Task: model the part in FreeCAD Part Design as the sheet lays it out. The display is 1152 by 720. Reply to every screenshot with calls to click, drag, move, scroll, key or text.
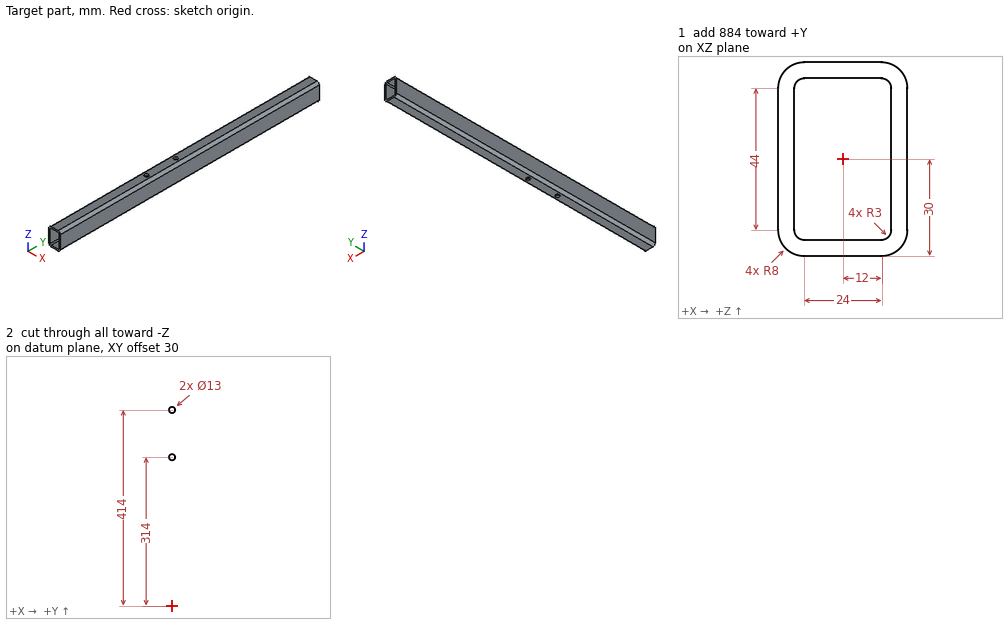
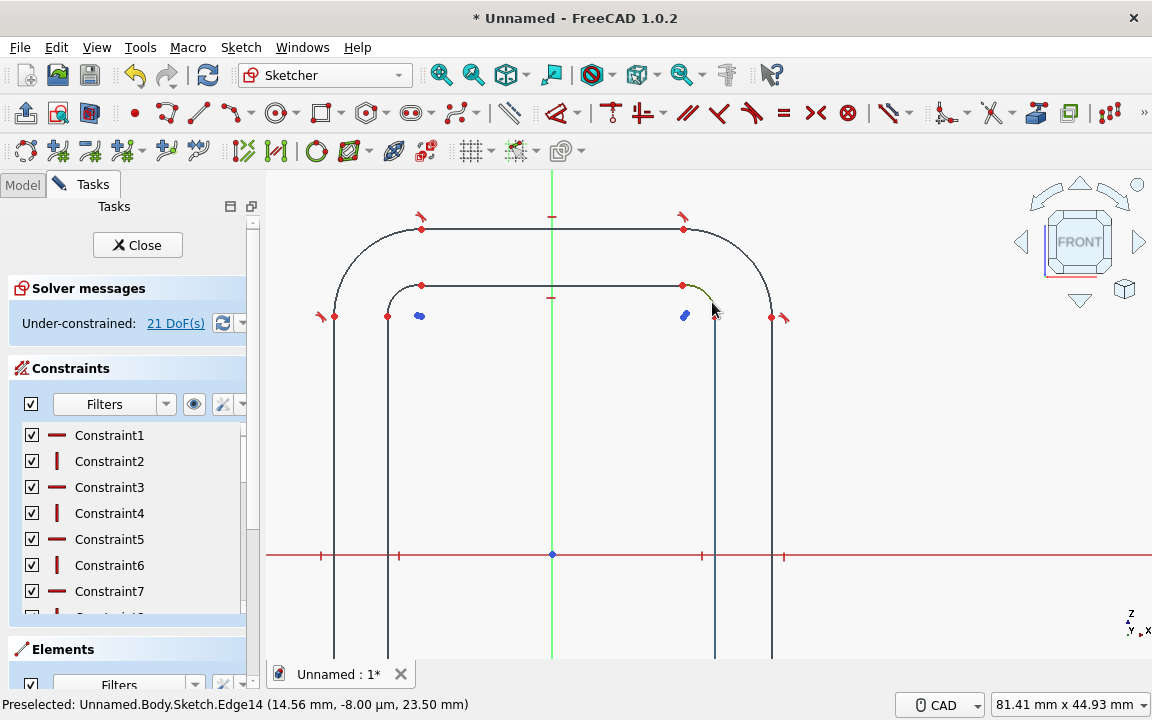
key(t)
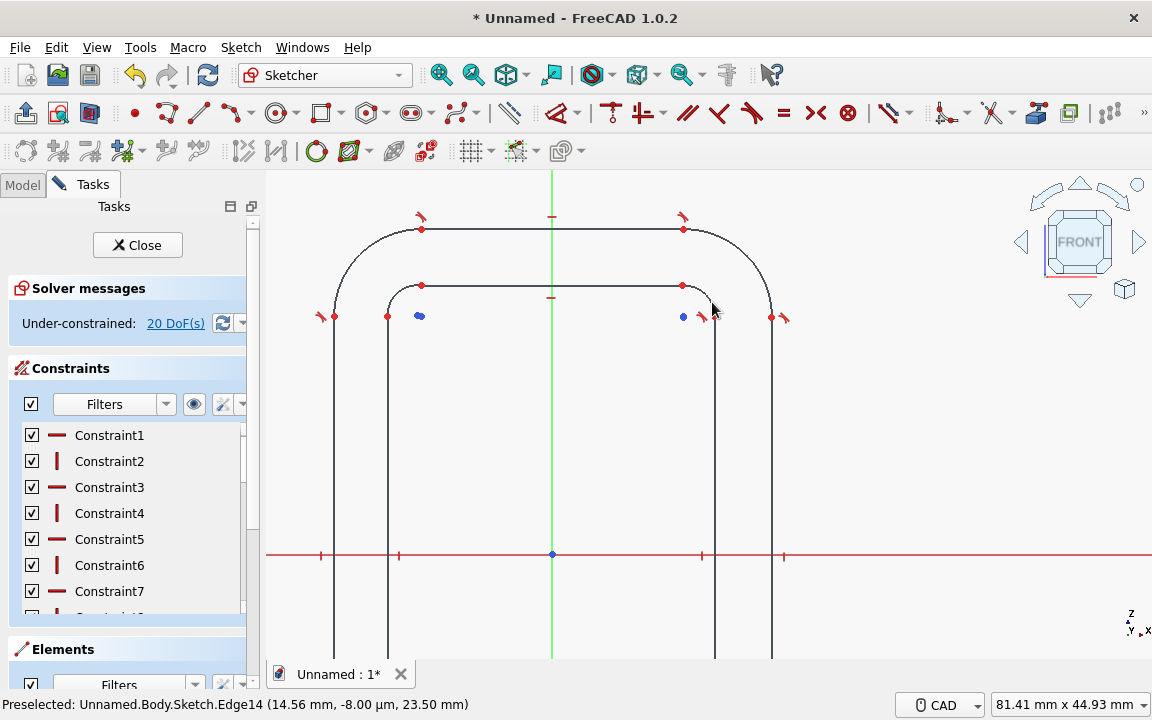
click(604, 286)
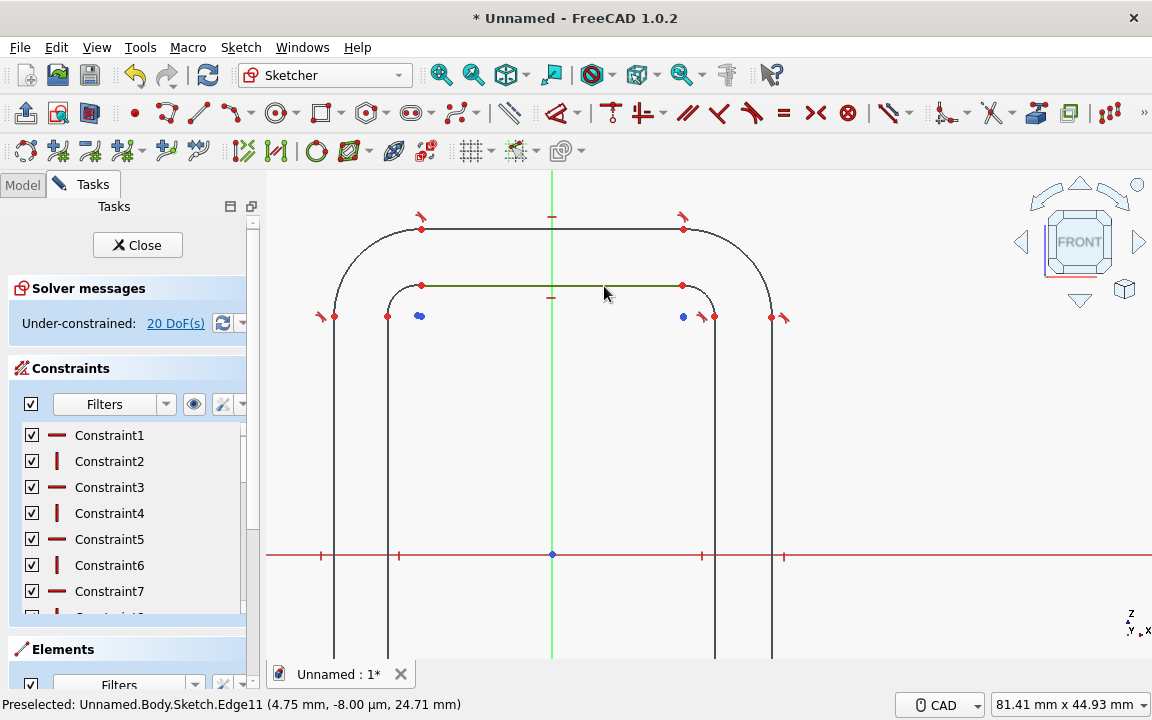
click(711, 302)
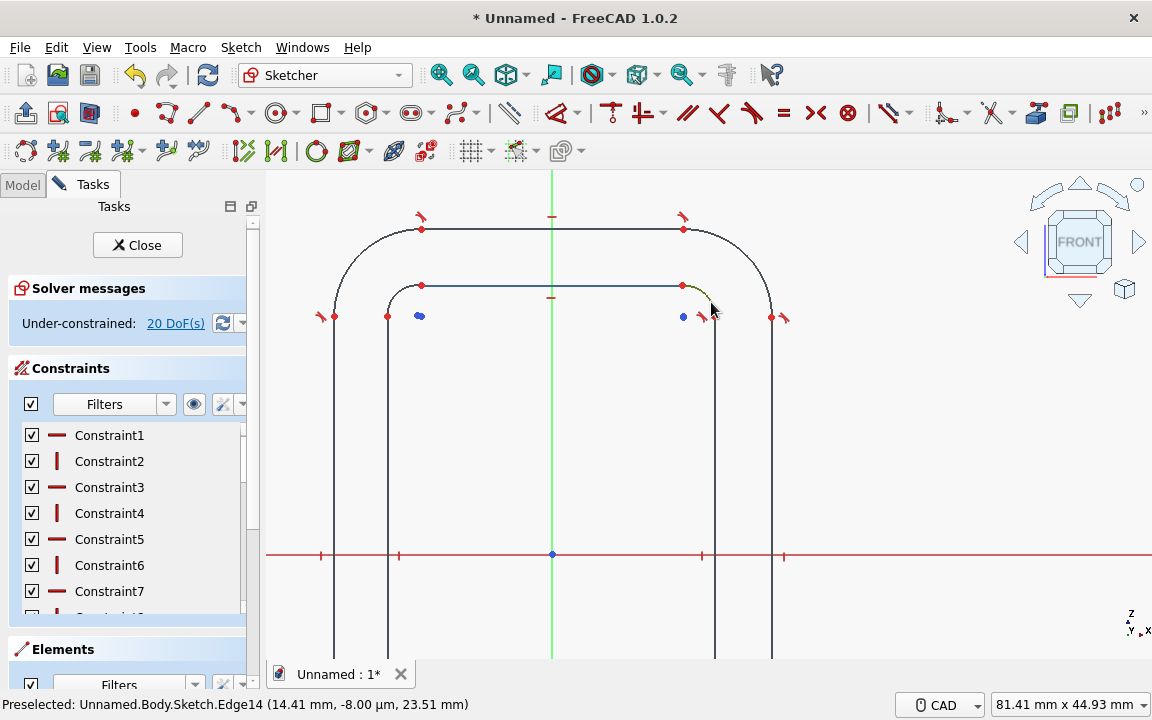
key(t)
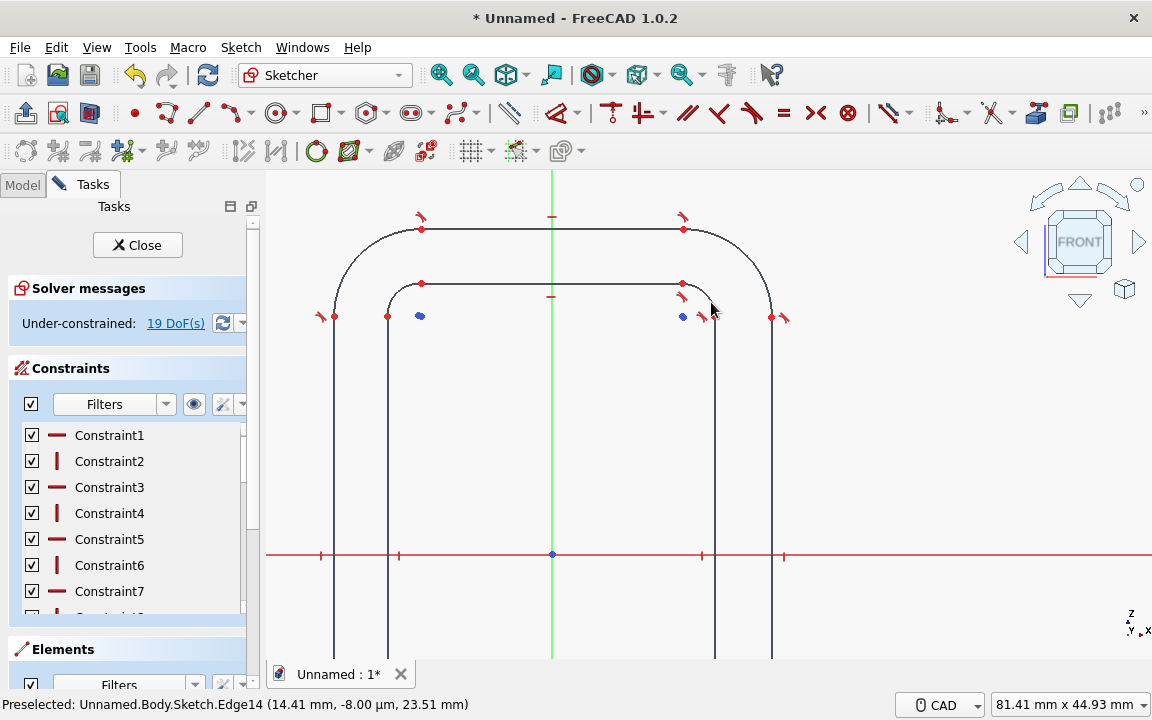
click(604, 284)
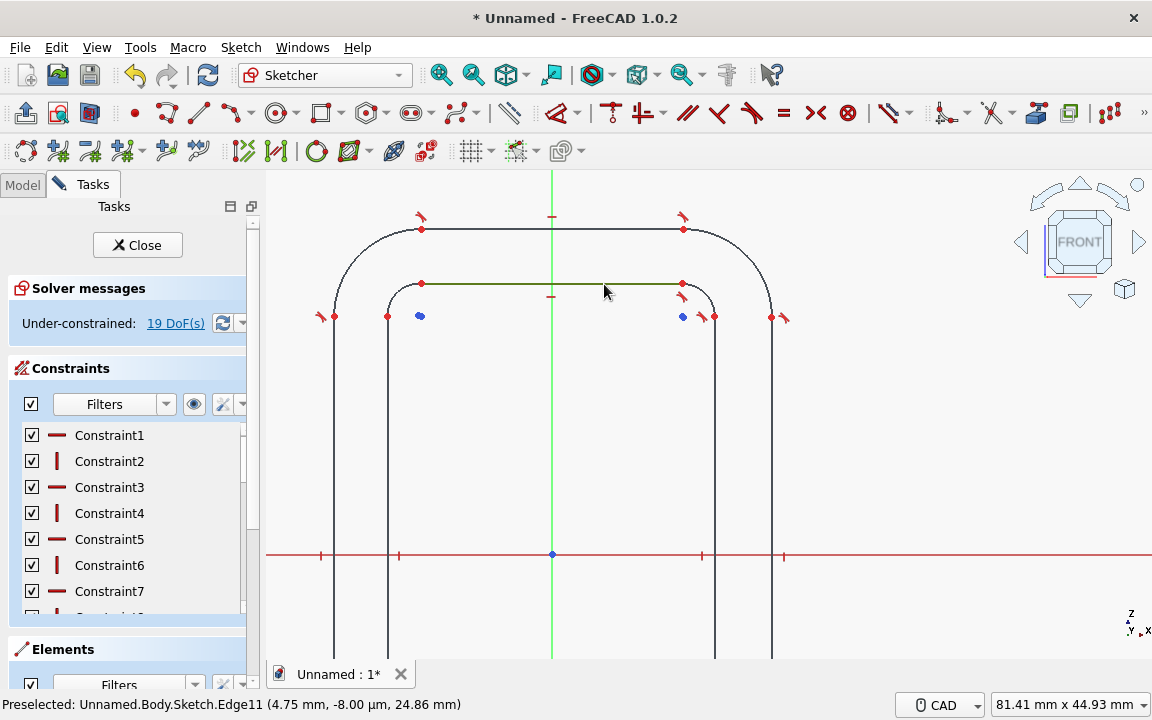
click(406, 287)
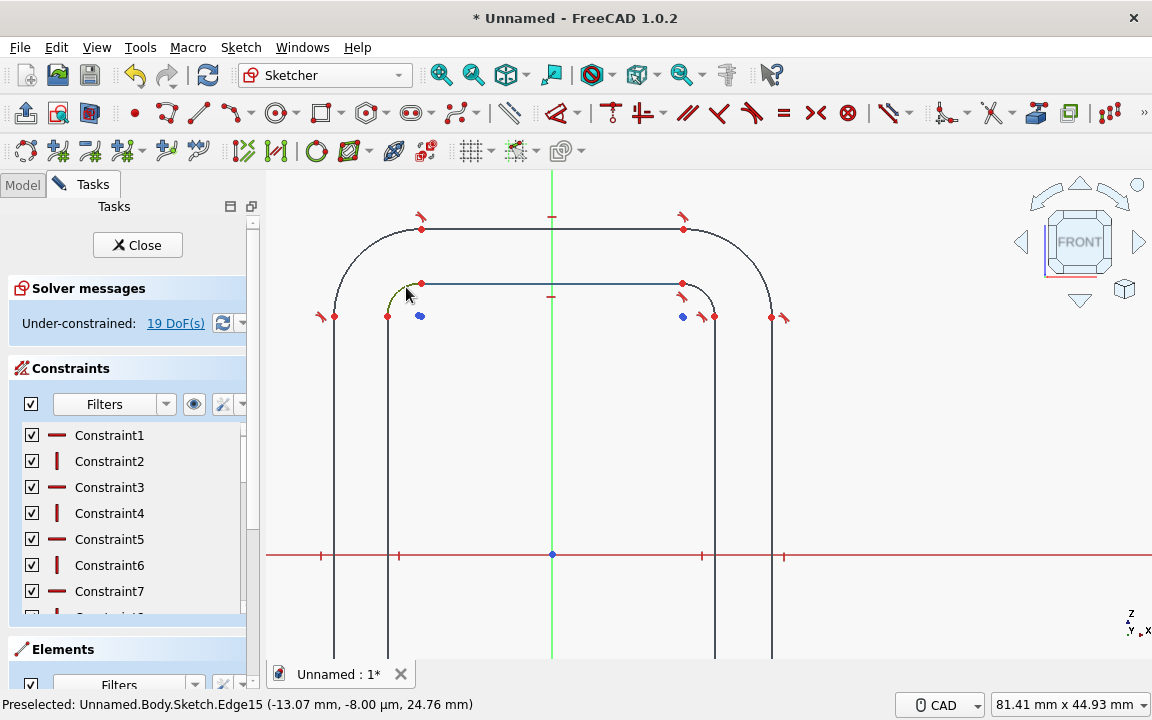
key(t)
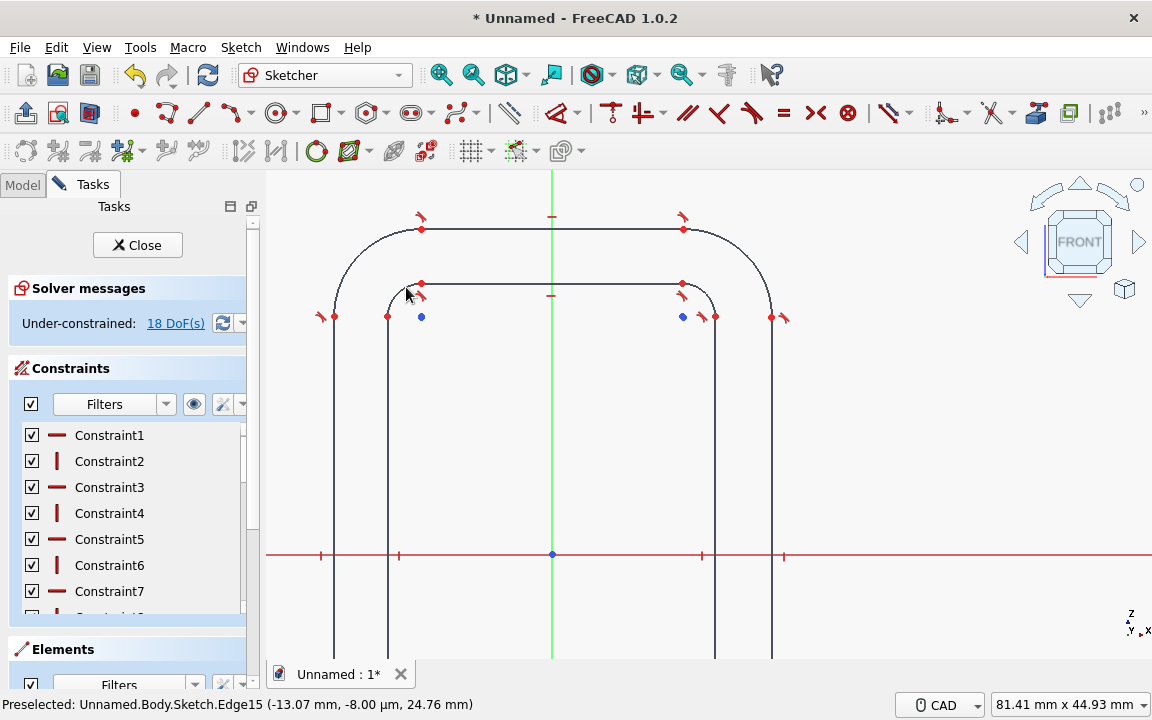
click(388, 460)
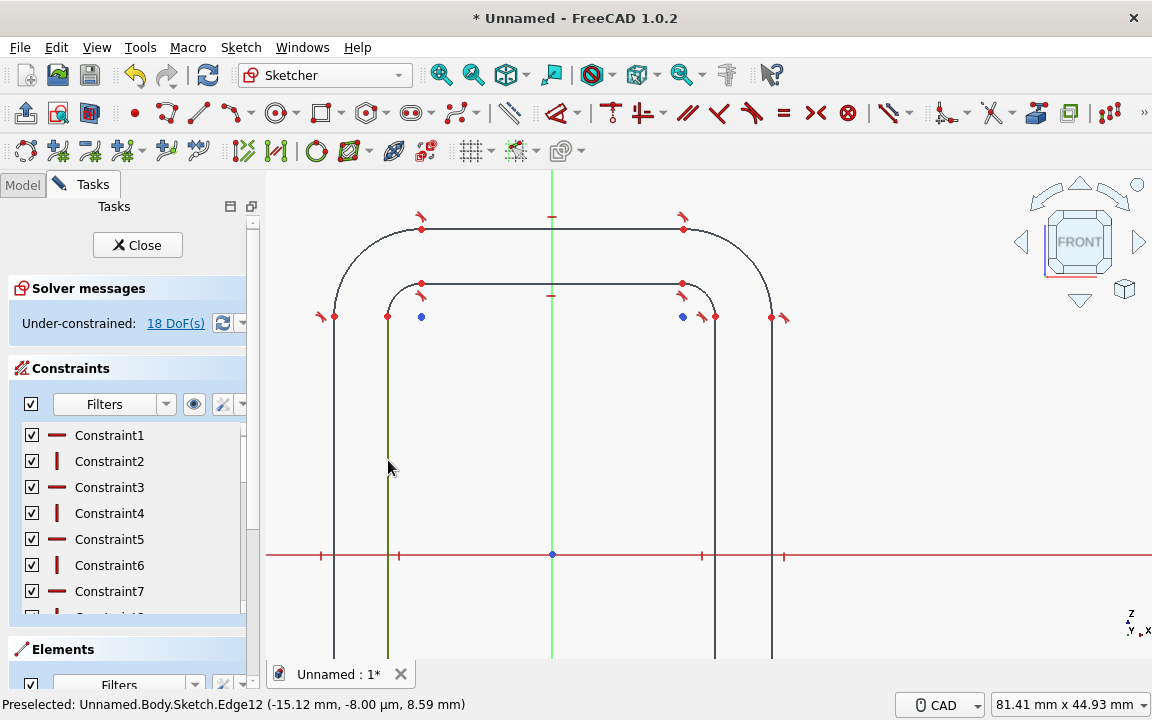
click(406, 287)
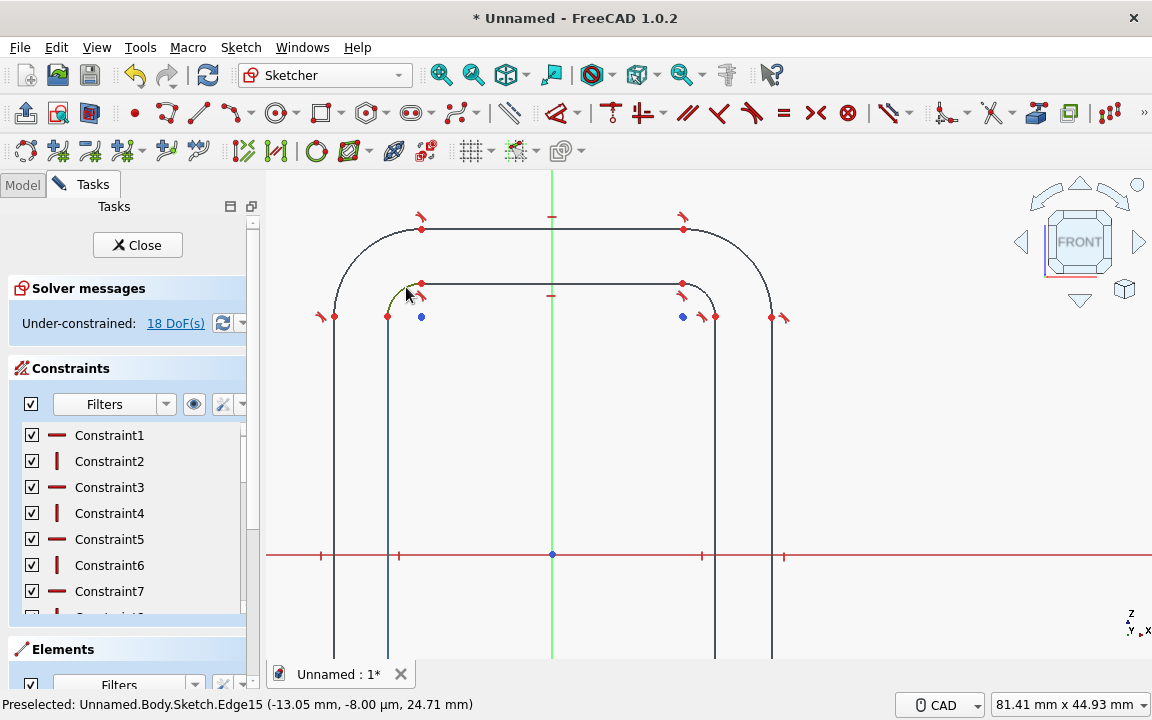
key(t)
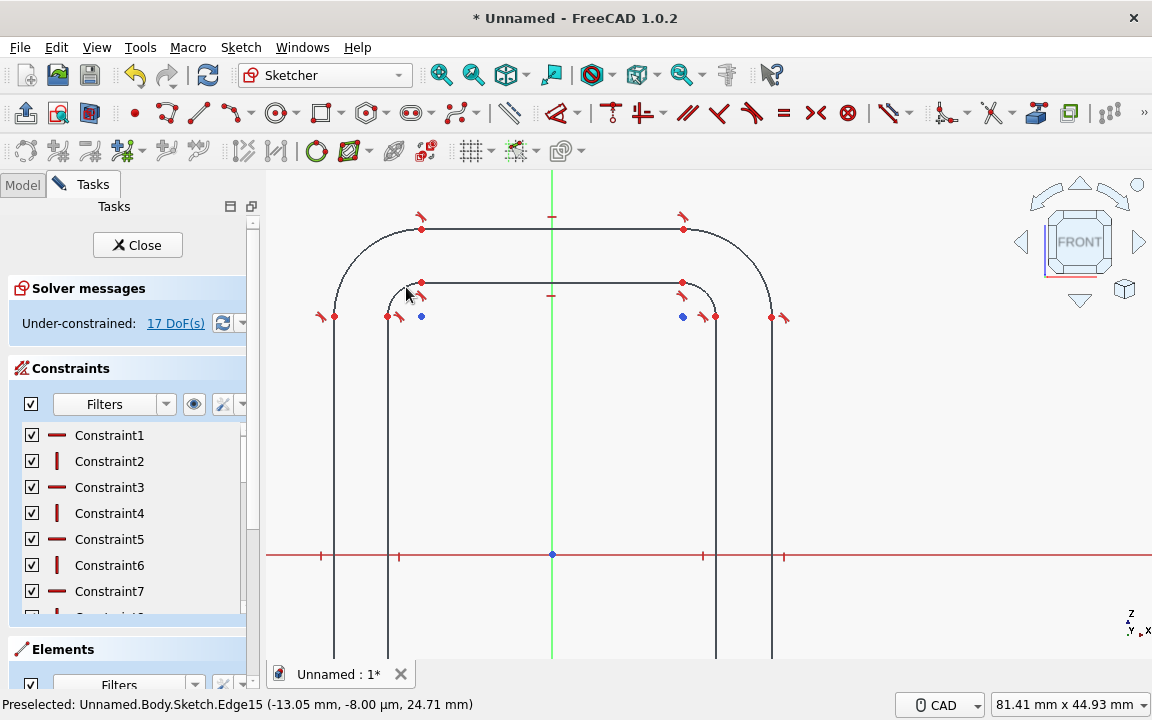
click(388, 460)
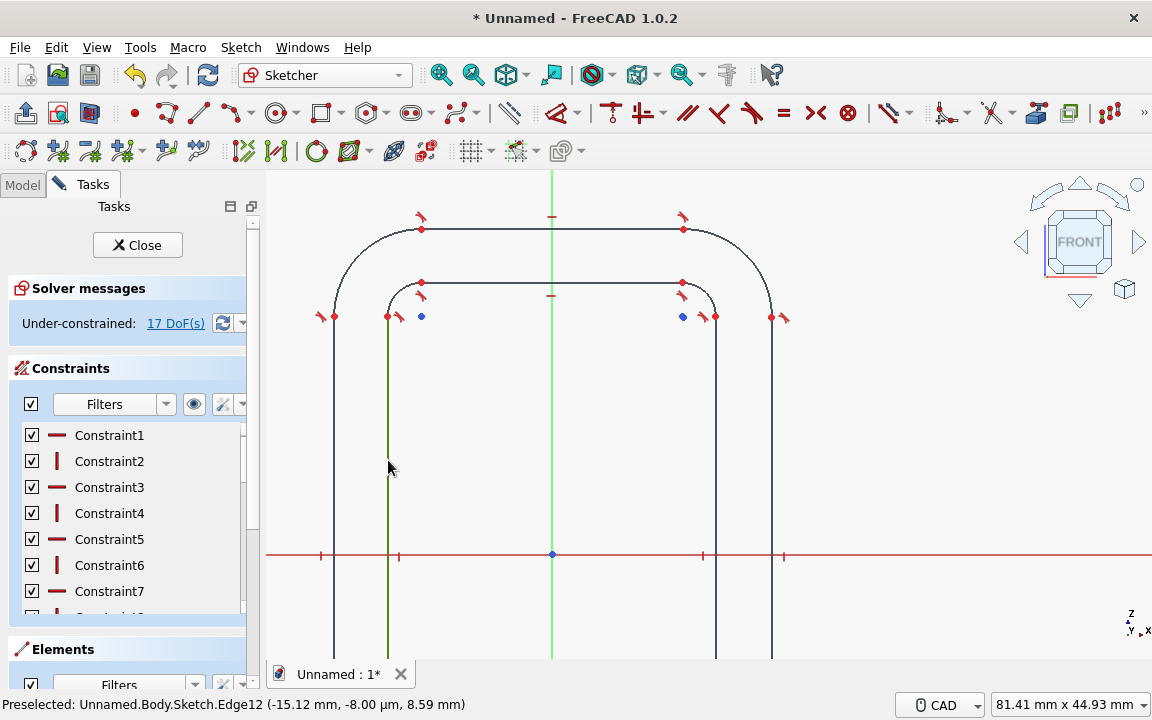
scroll(713, 300, down, 4)